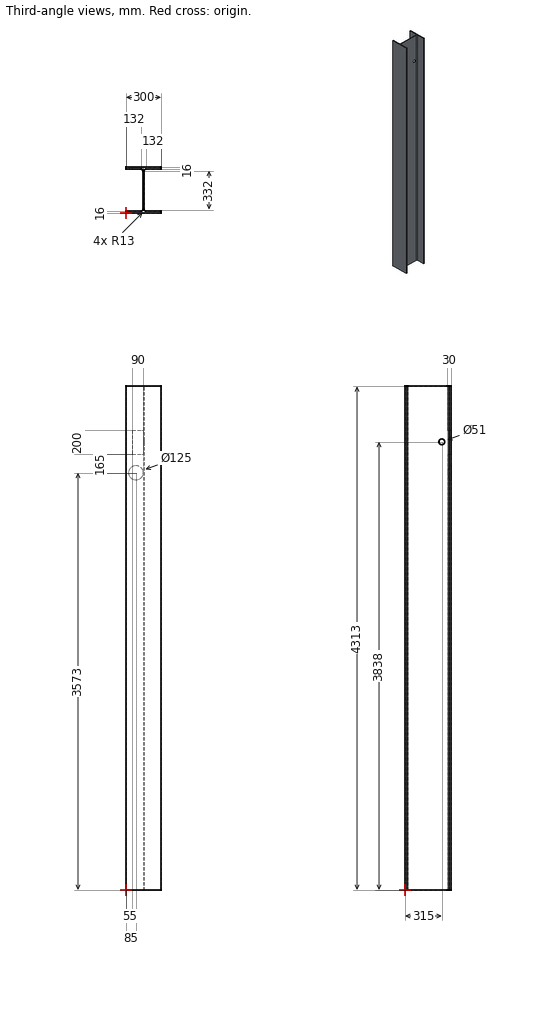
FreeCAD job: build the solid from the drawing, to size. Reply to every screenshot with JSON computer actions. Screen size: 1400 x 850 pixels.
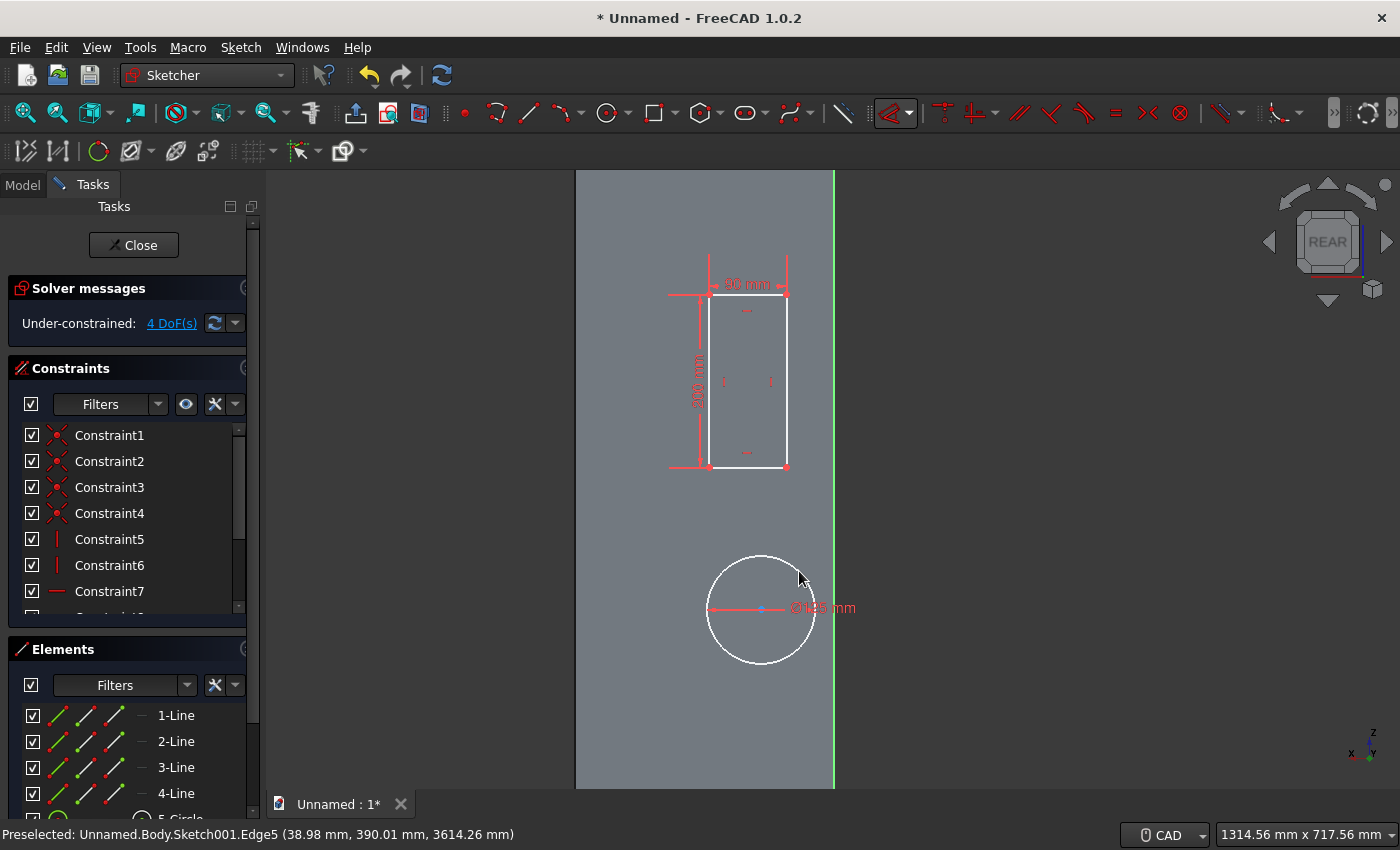
{"action": "left_click", "coordinate": [761, 610]}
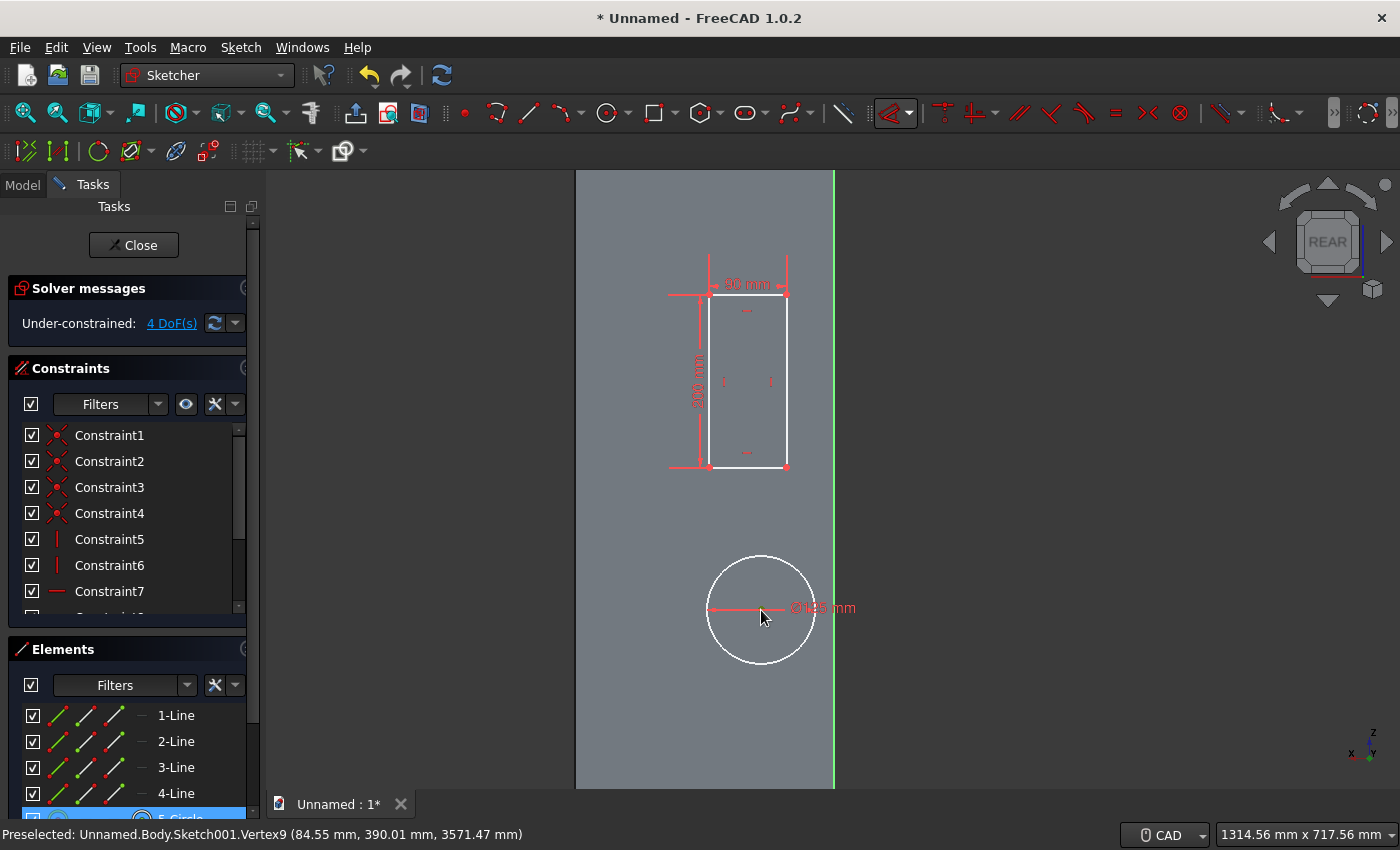
{"action": "left_click", "coordinate": [912, 114]}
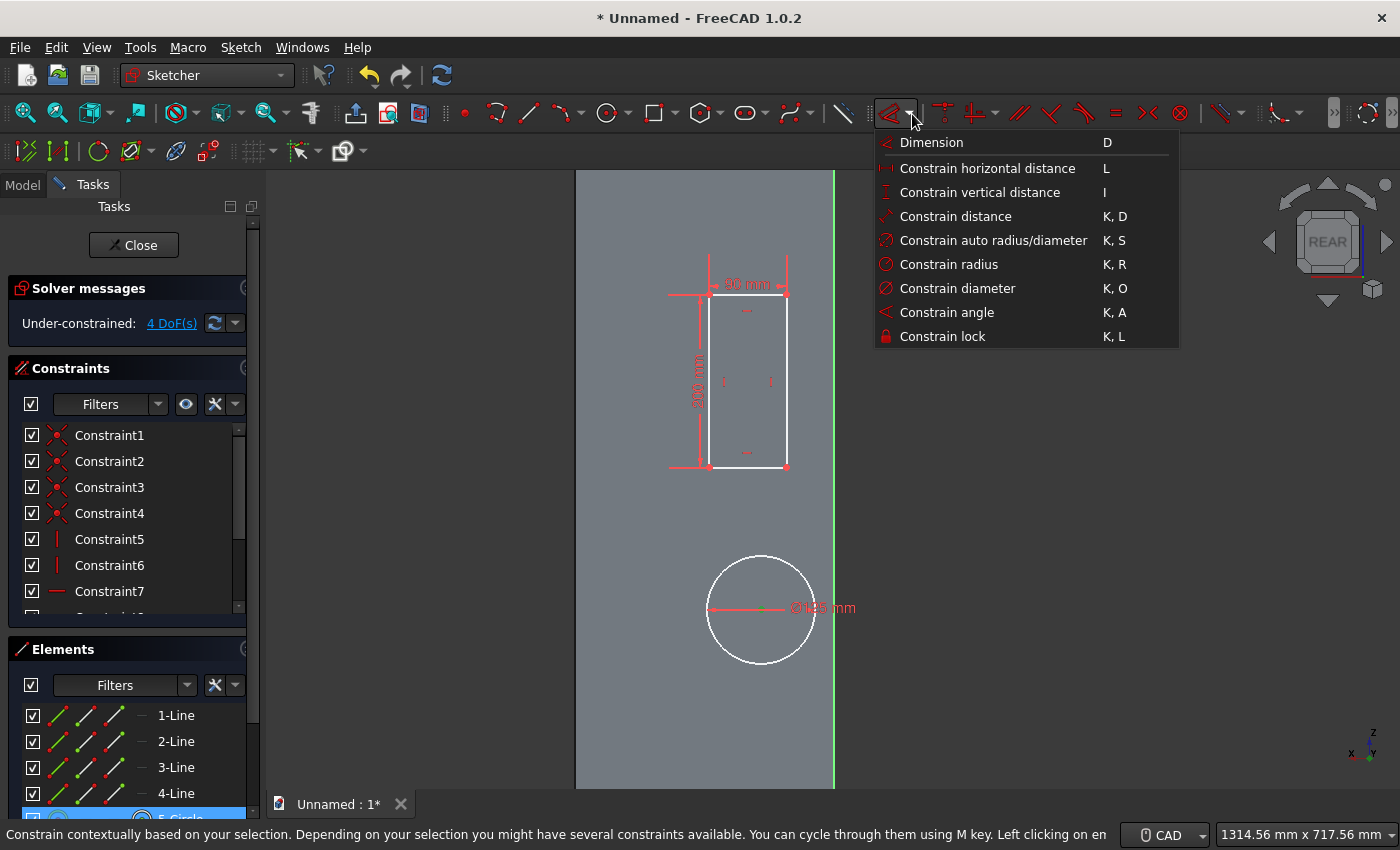
{"action": "left_click", "coordinate": [1027, 168]}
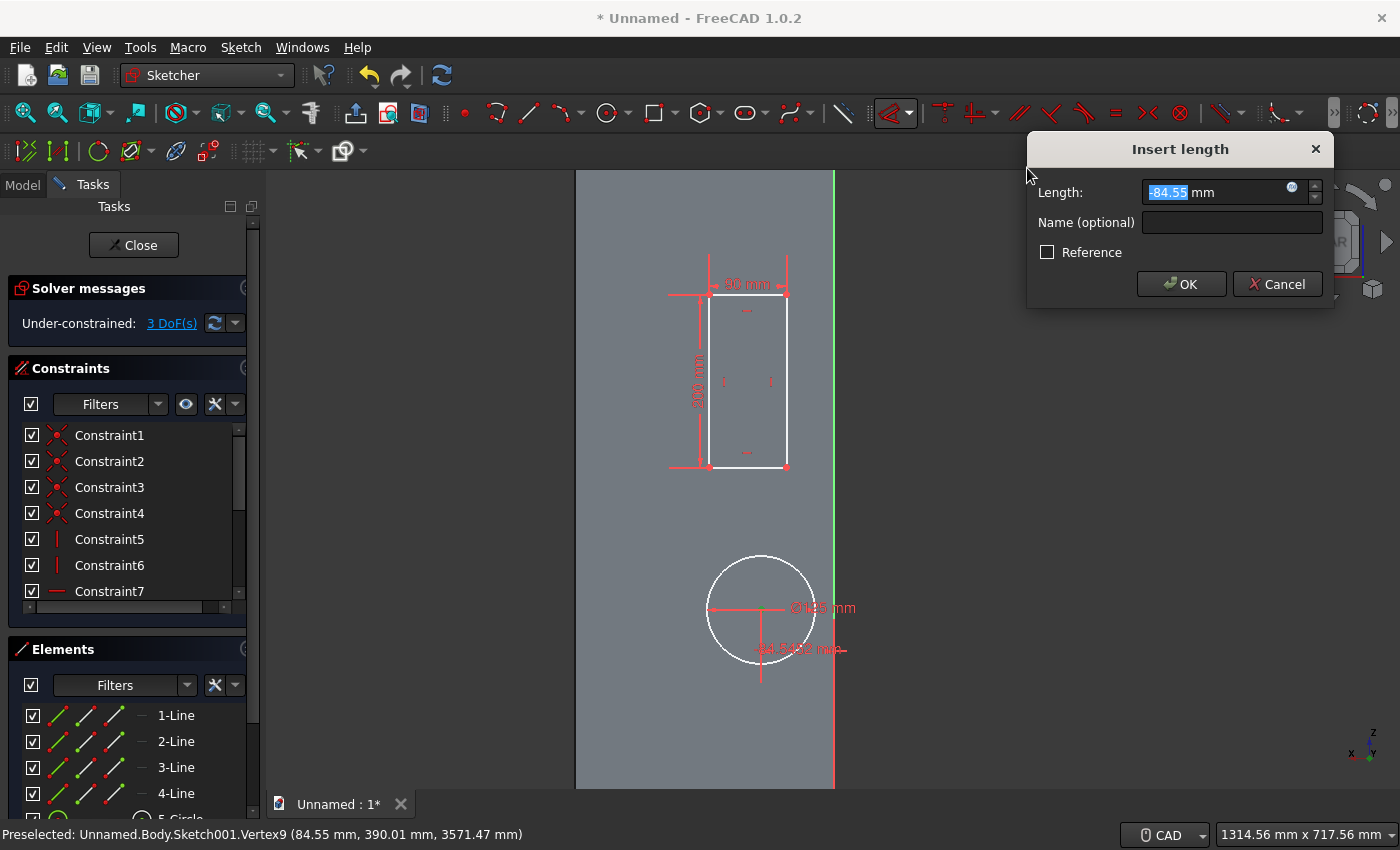
{"action": "type", "text": "-85"}
{"action": "key", "text": "Return"}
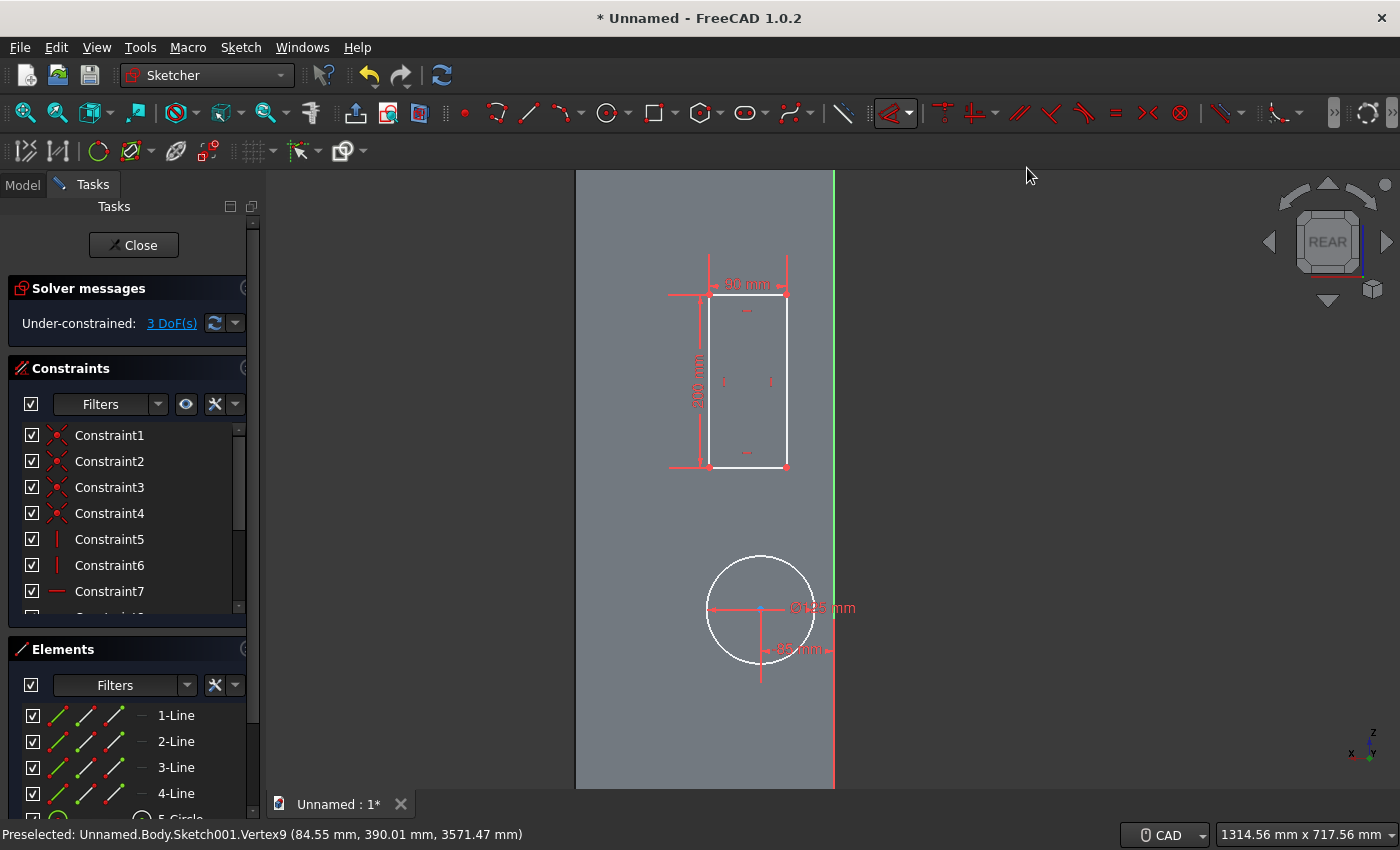
{"action": "left_click", "coordinate": [787, 468]}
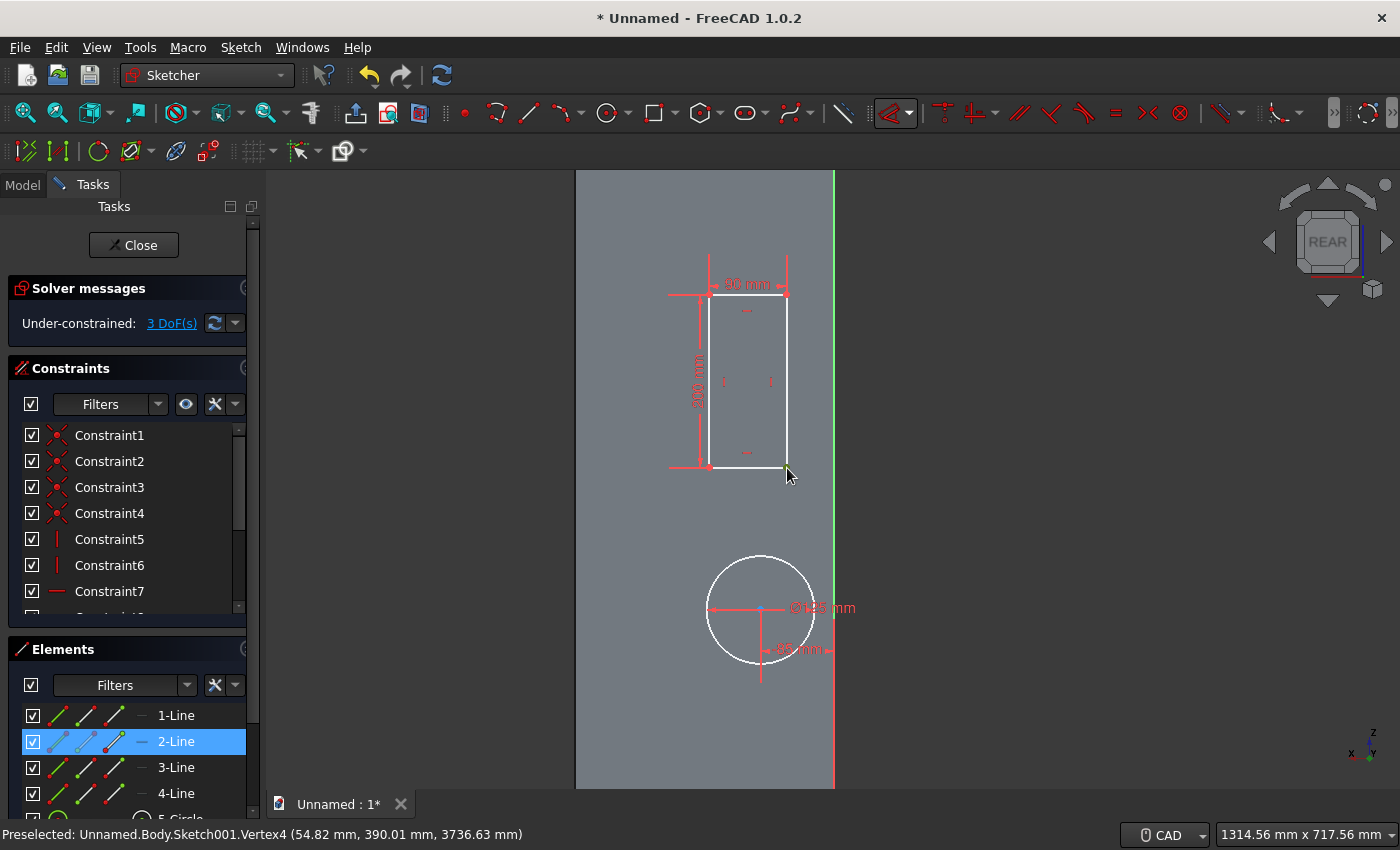
{"action": "left_click", "coordinate": [912, 114]}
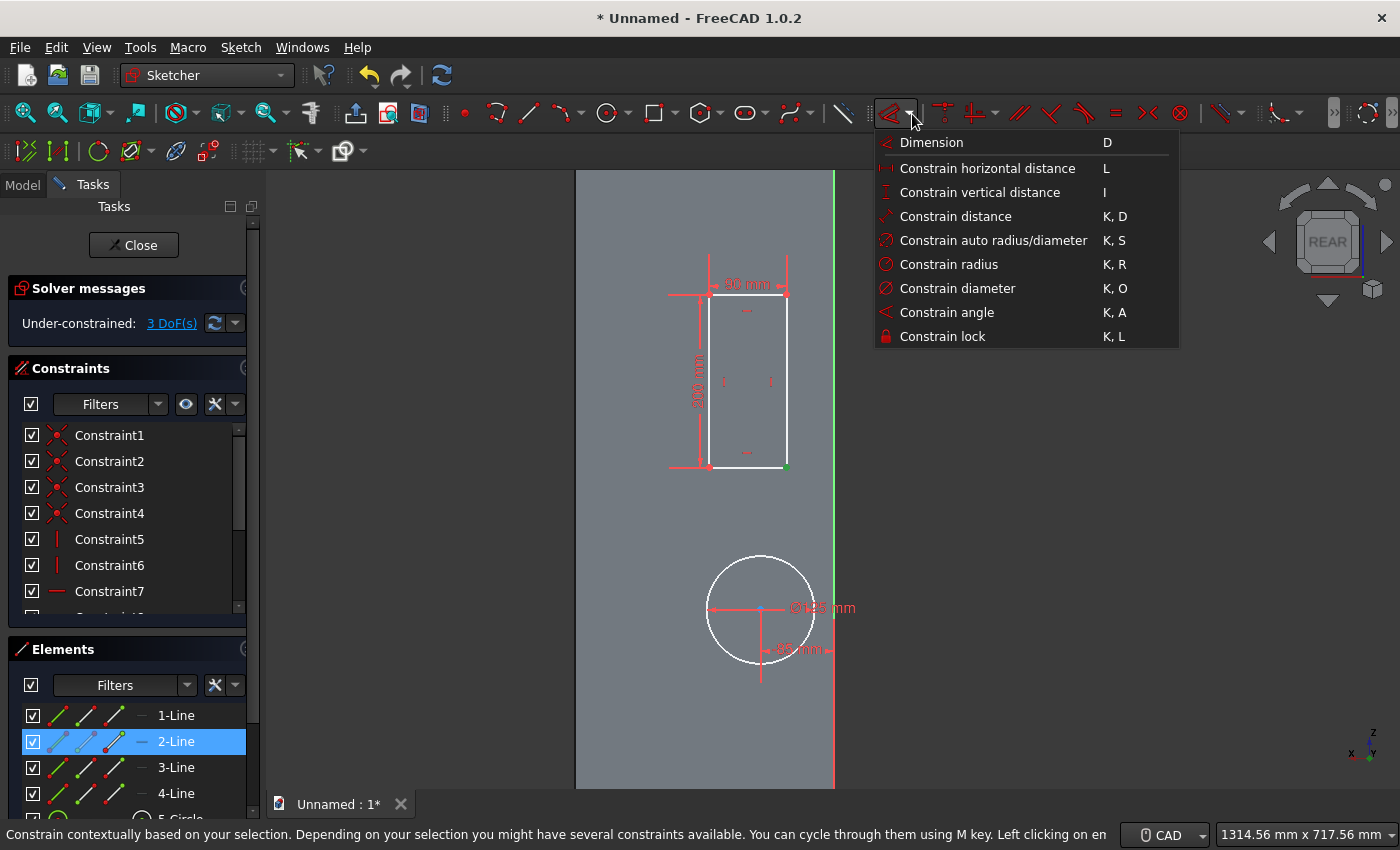
{"action": "left_click", "coordinate": [1027, 168]}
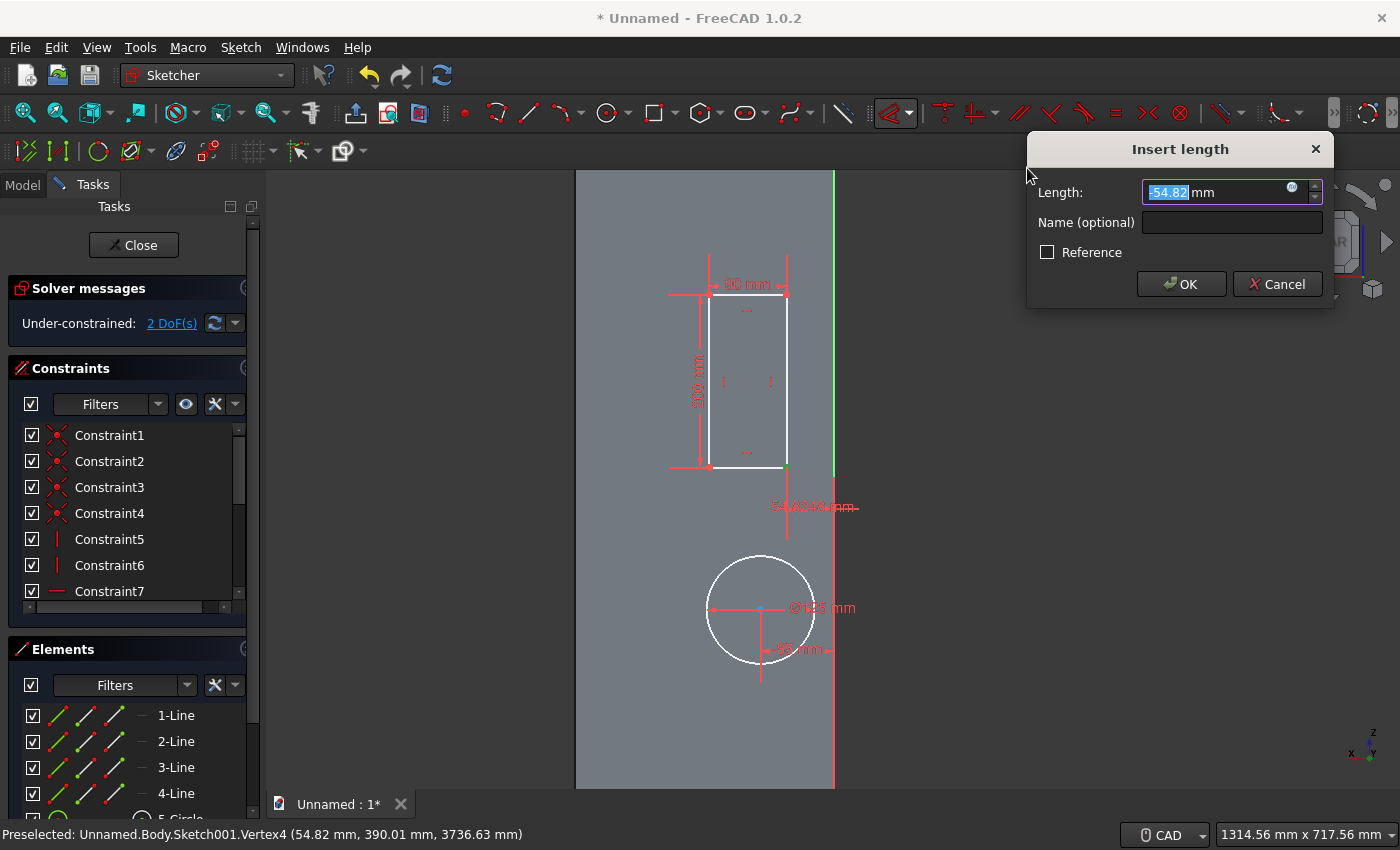
{"action": "type", "text": "-55"}
{"action": "key", "text": "Return"}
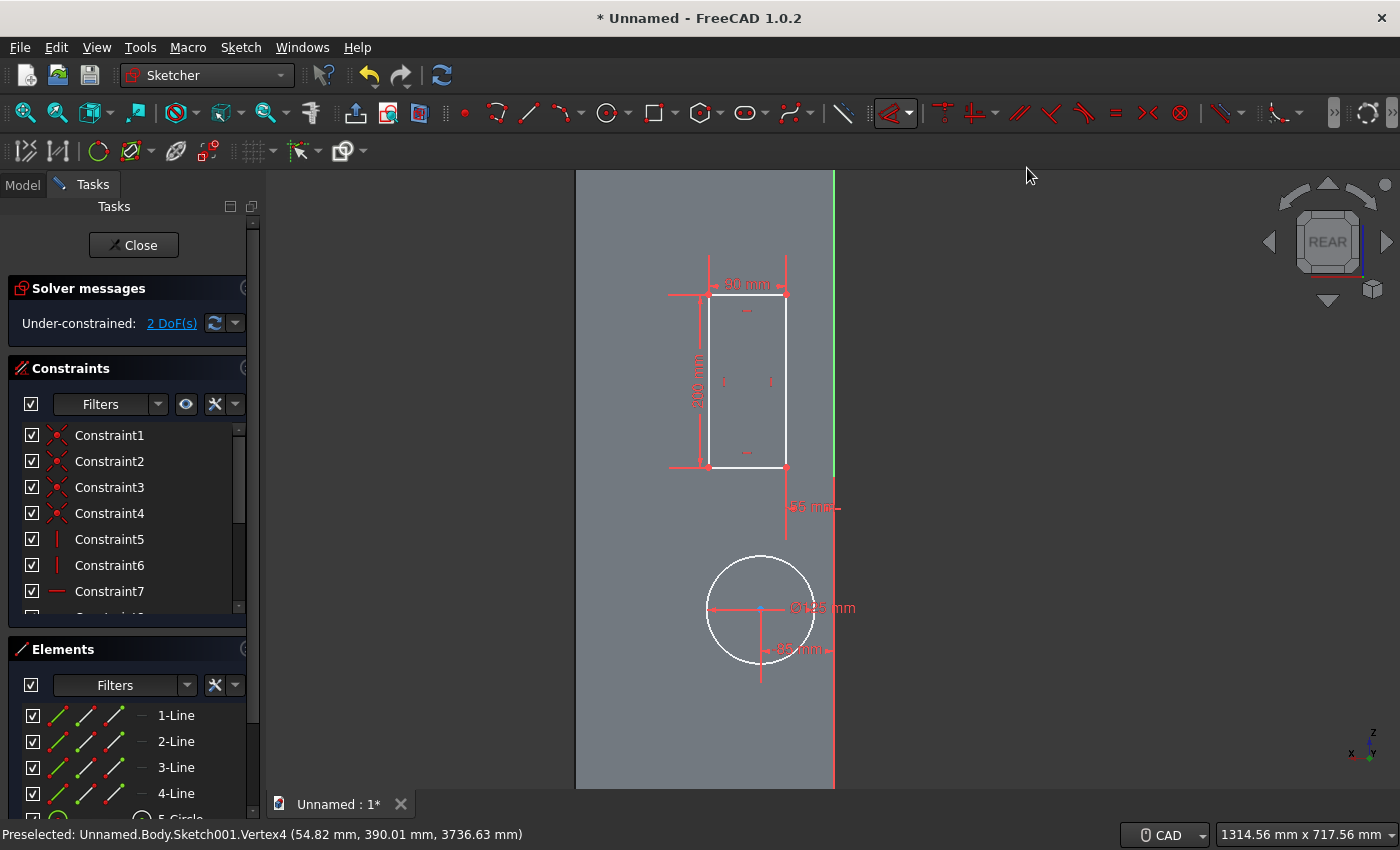
{"action": "left_click", "coordinate": [761, 610]}